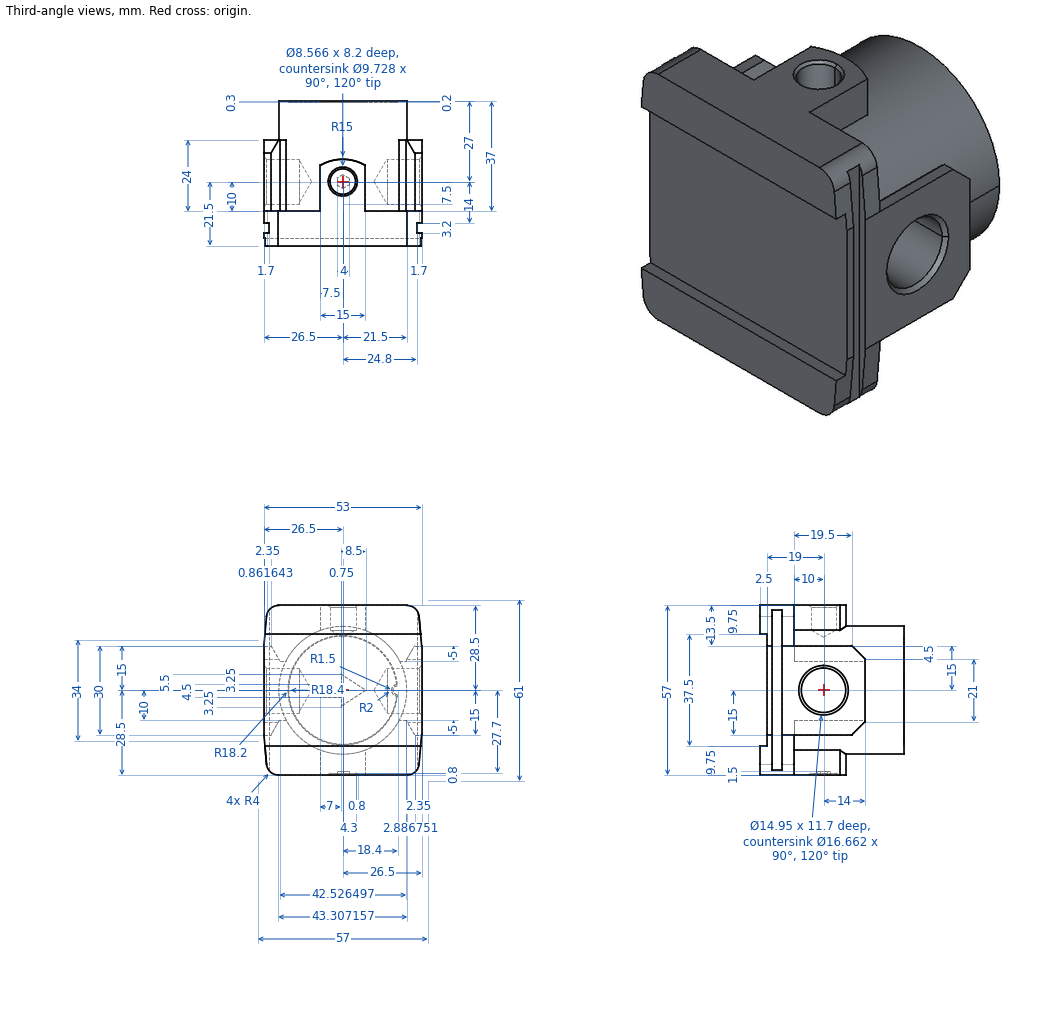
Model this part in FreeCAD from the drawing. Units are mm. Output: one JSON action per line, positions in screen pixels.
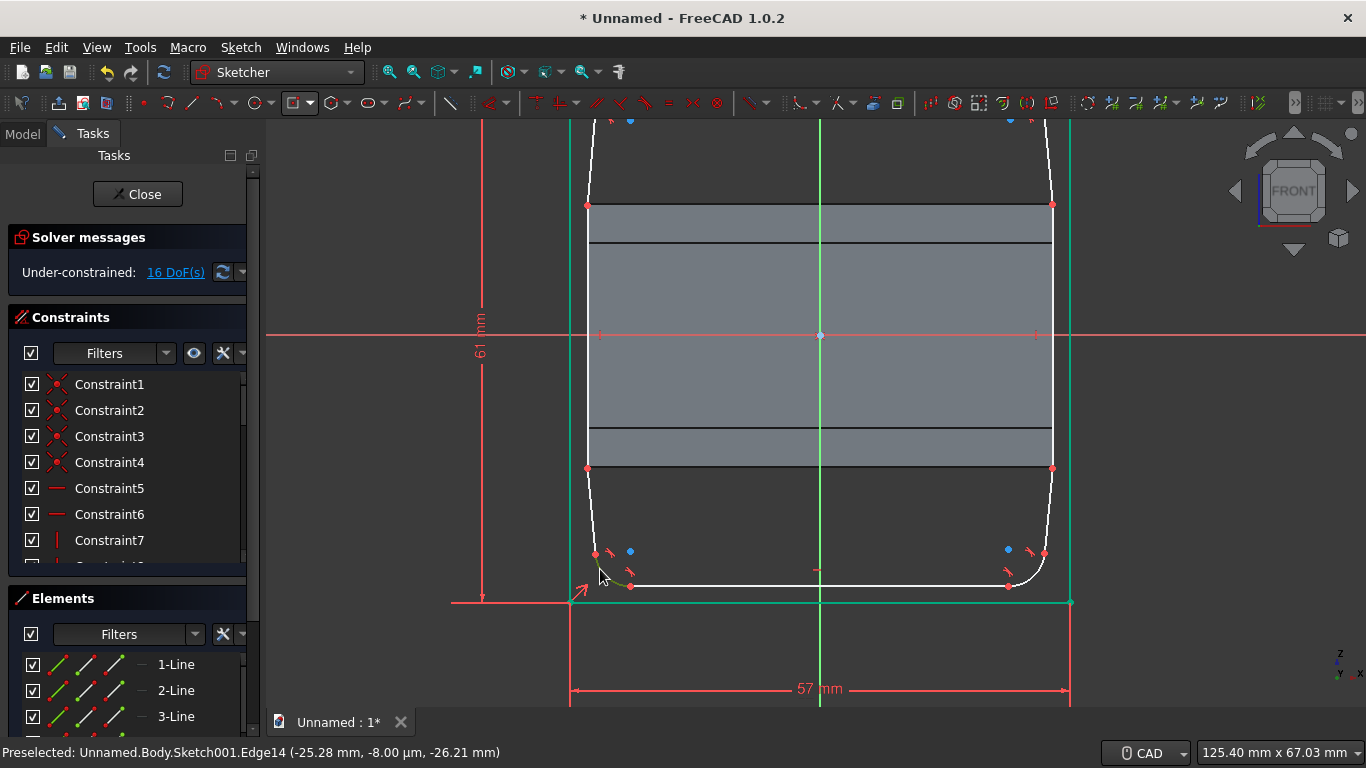
{"action": "left_click", "coordinate": [1024, 583]}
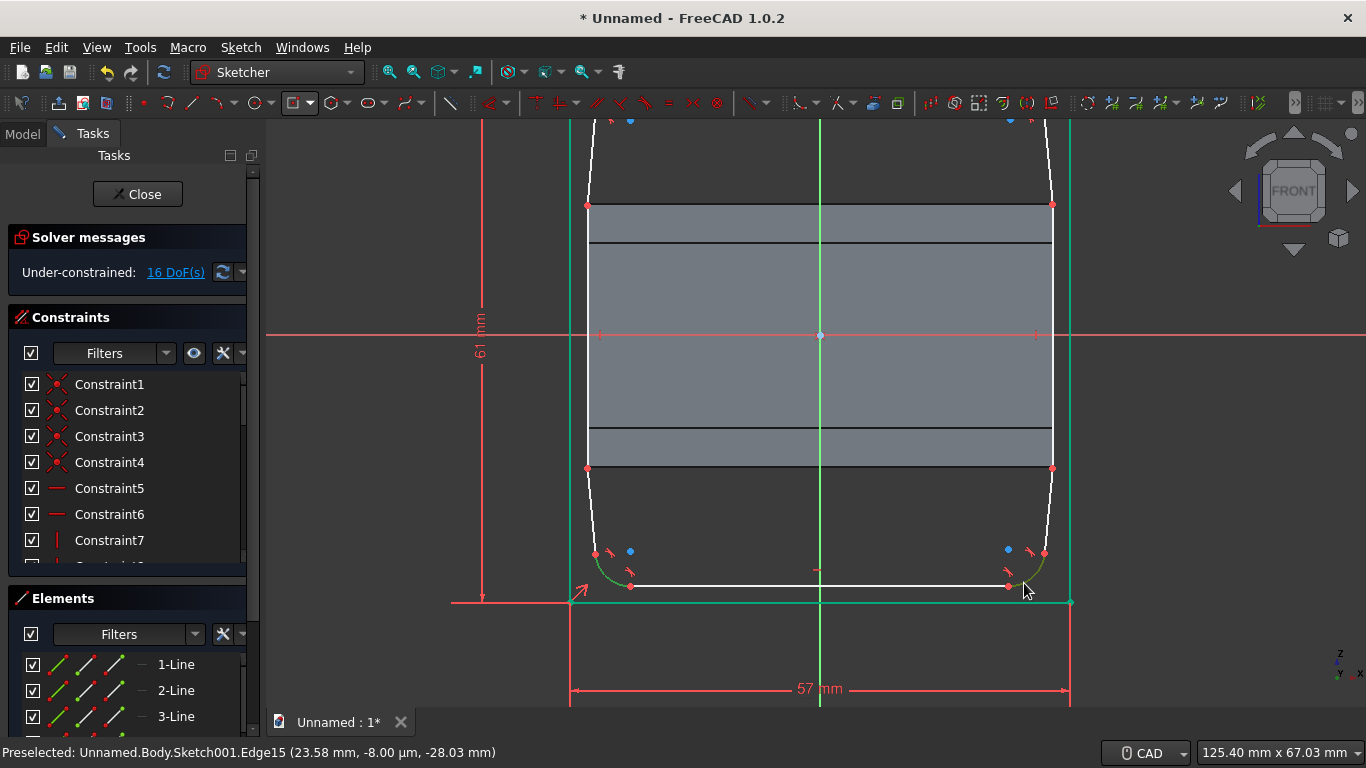
{"action": "scroll", "coordinate": [600, 571], "scroll_direction": "down", "scroll_amount": 2}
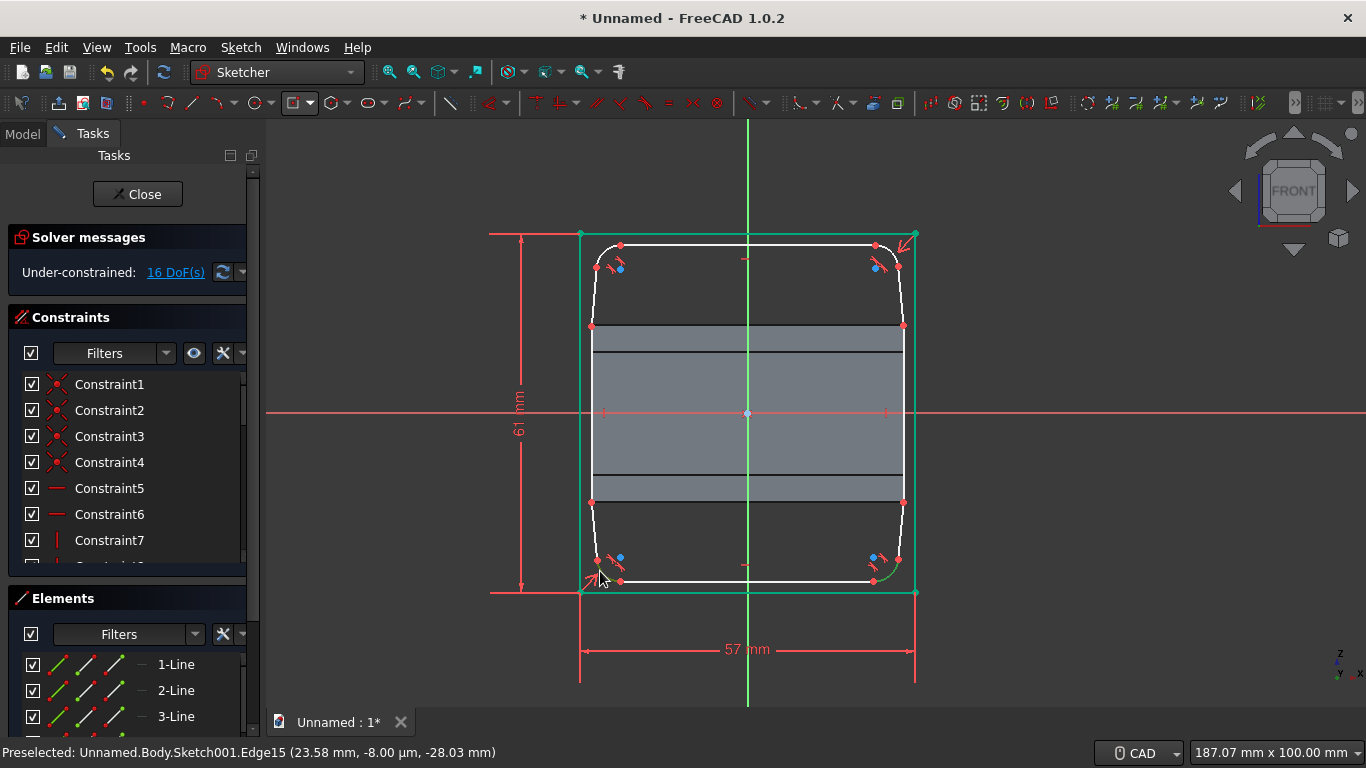
{"action": "scroll", "coordinate": [895, 257], "scroll_direction": "up", "scroll_amount": 2}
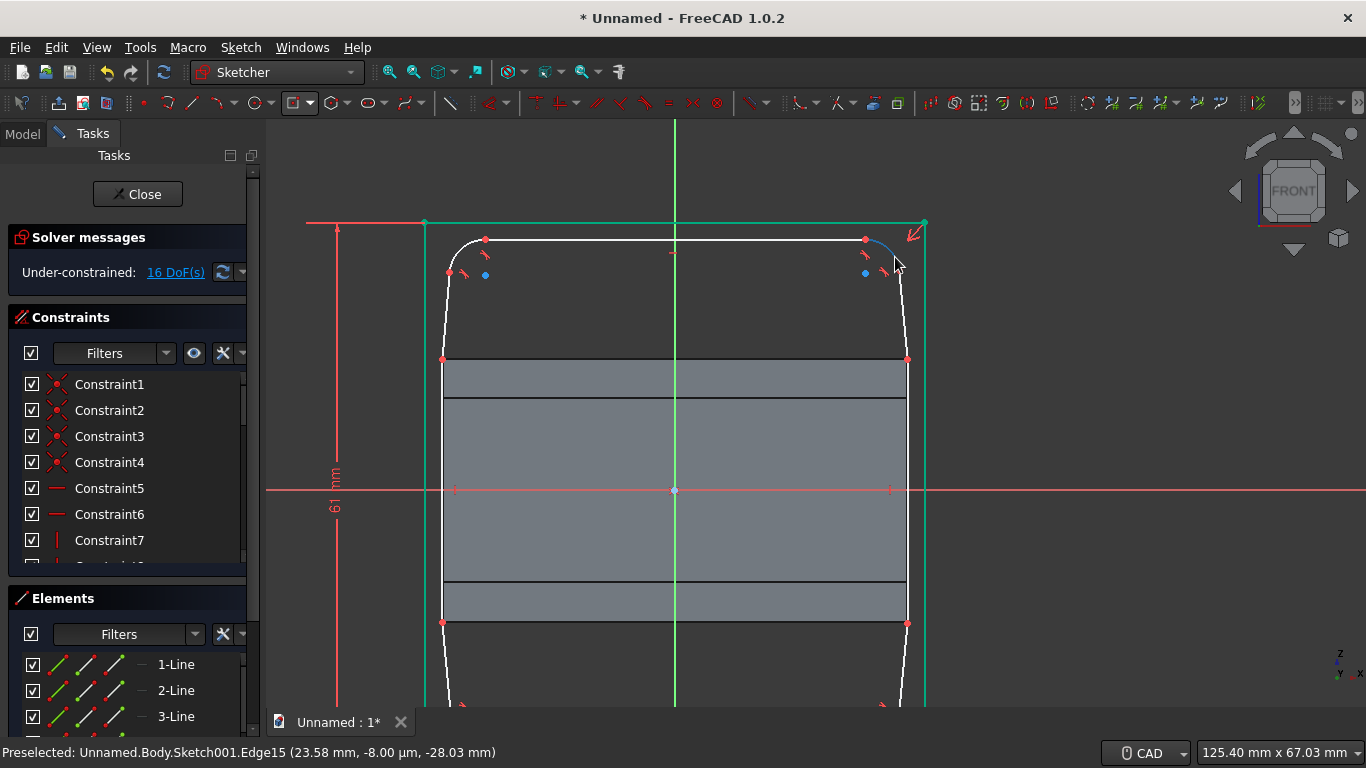
{"action": "left_click", "coordinate": [895, 256]}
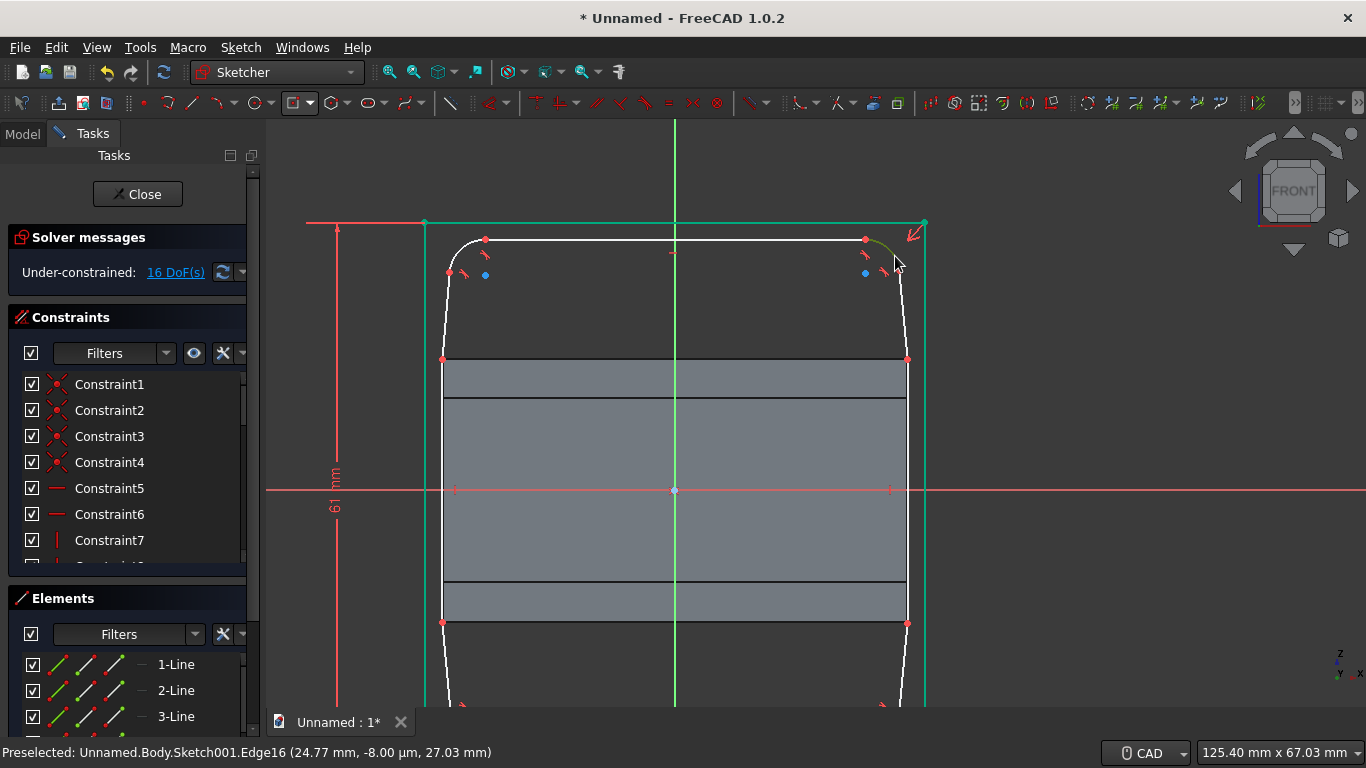
{"action": "left_click", "coordinate": [470, 243]}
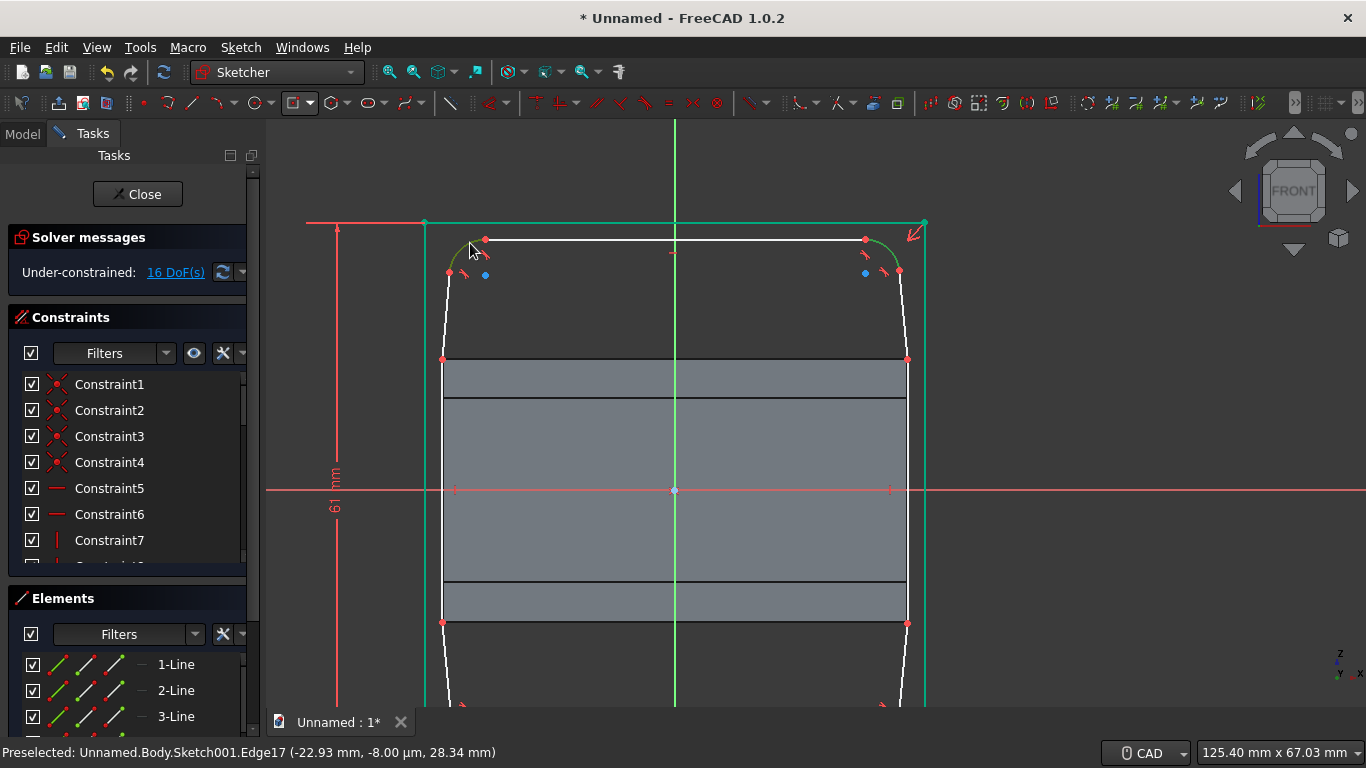
{"action": "left_click", "coordinate": [670, 104]}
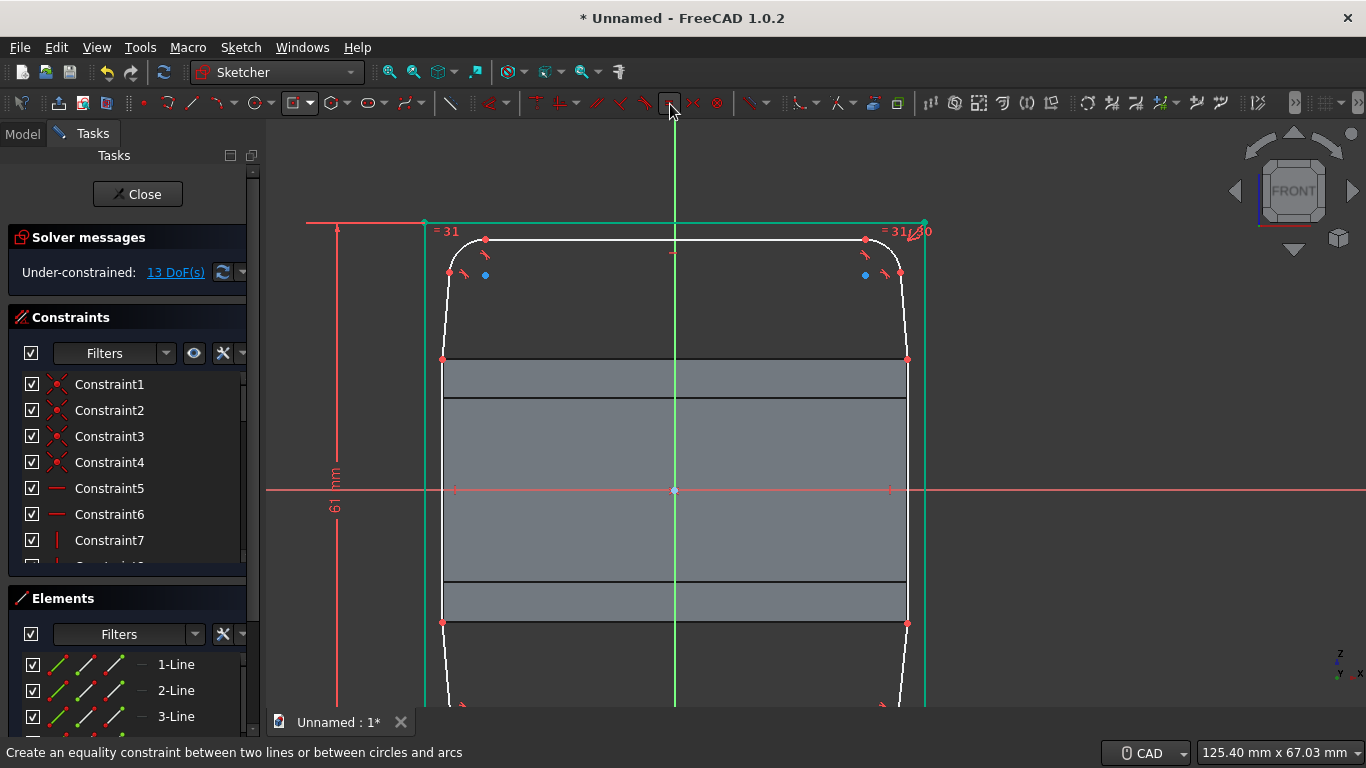
{"action": "left_click", "coordinate": [490, 104]}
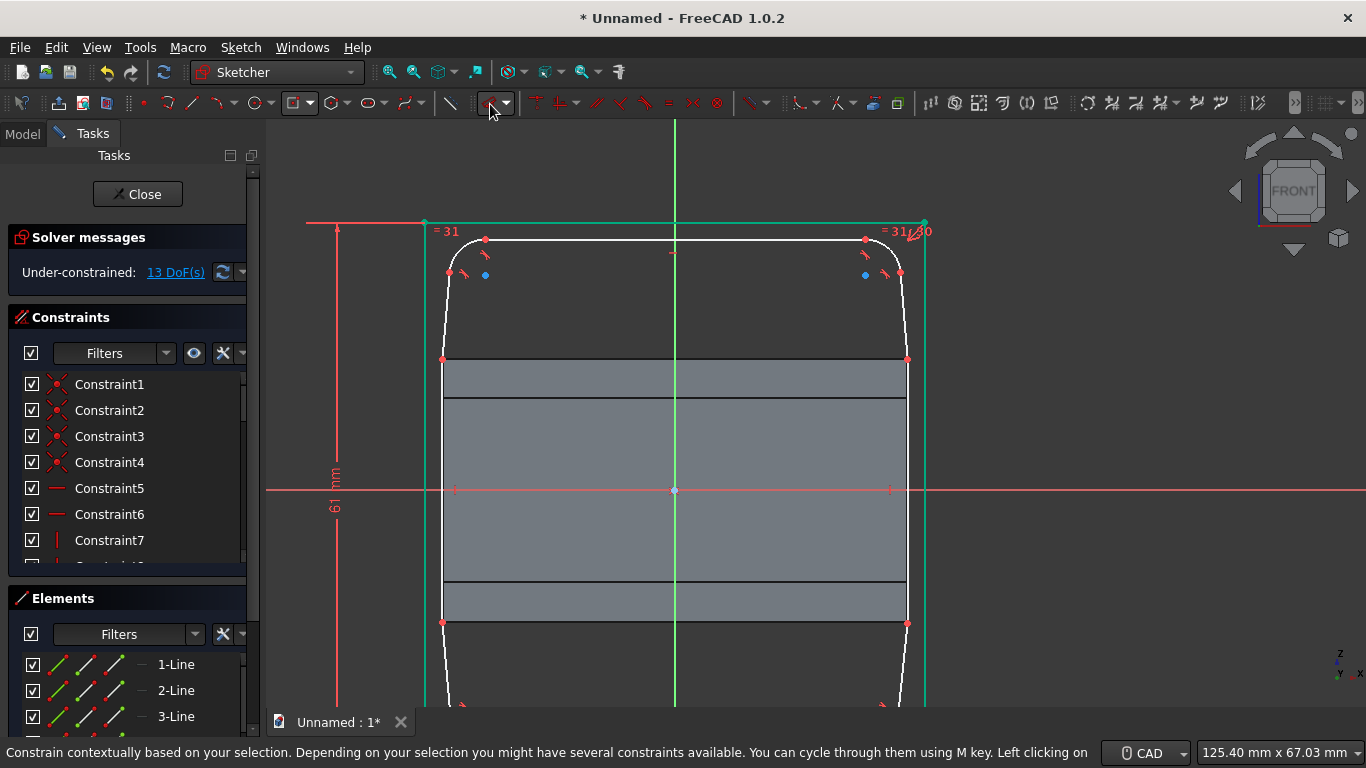
{"action": "scroll", "coordinate": [895, 256], "scroll_direction": "down", "scroll_amount": 2}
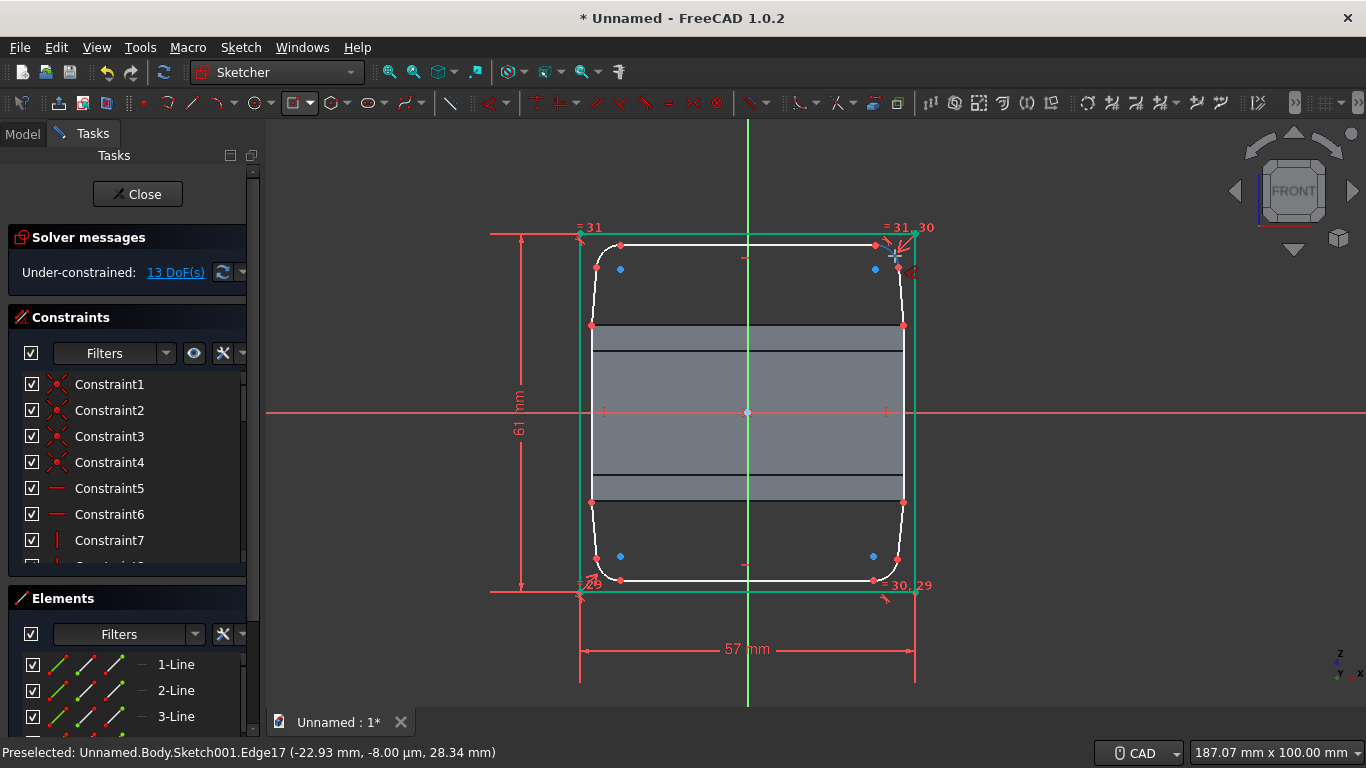
{"action": "scroll", "coordinate": [600, 569], "scroll_direction": "up", "scroll_amount": 3}